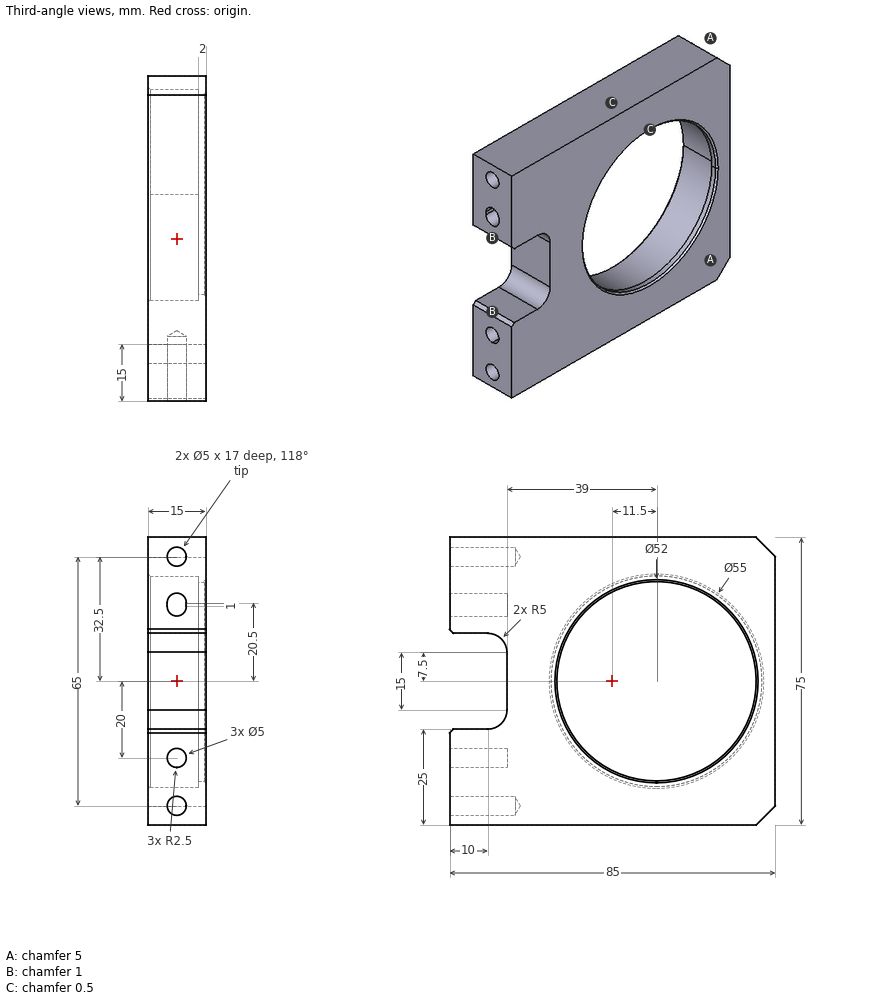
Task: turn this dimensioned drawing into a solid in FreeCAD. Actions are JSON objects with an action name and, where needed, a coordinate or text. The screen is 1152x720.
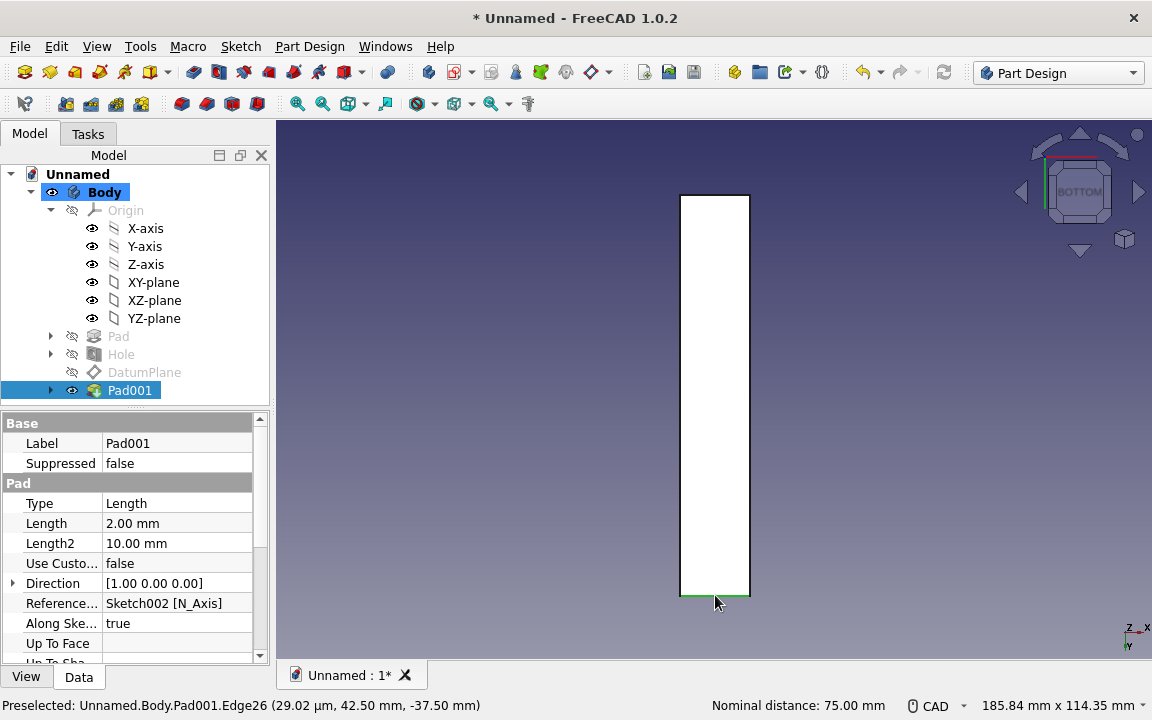
{"action": "left_click", "coordinate": [207, 104]}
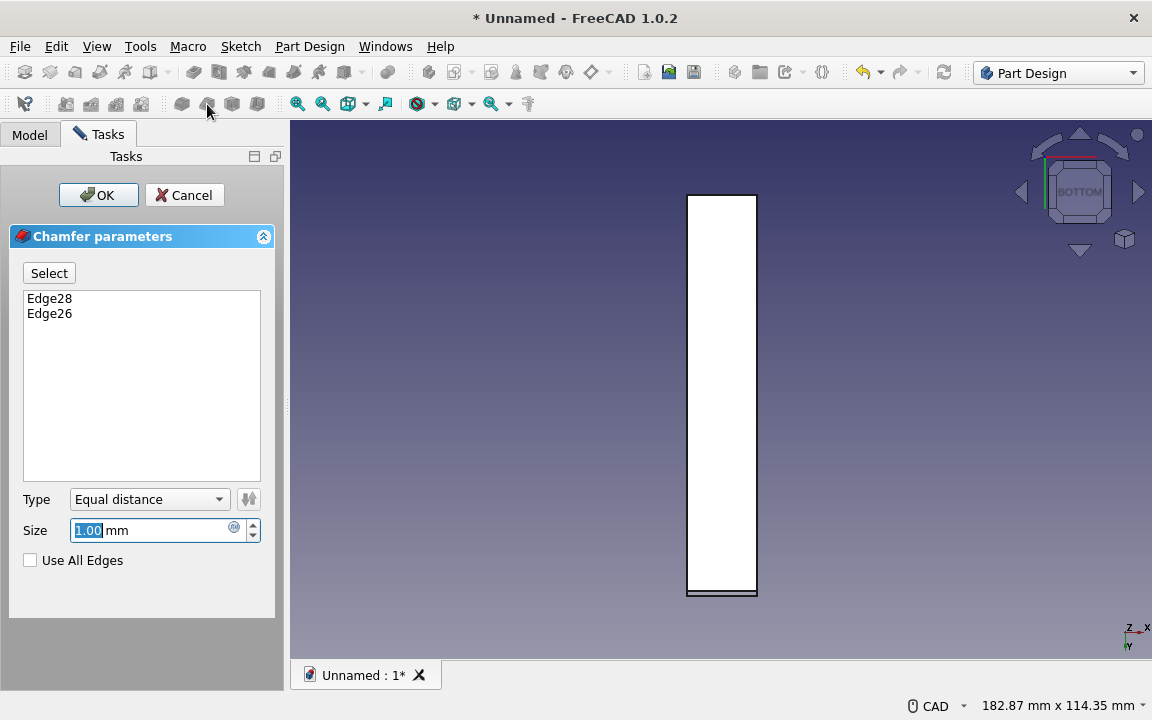
{"action": "type", "text": "5"}
{"action": "key", "text": "Tab"}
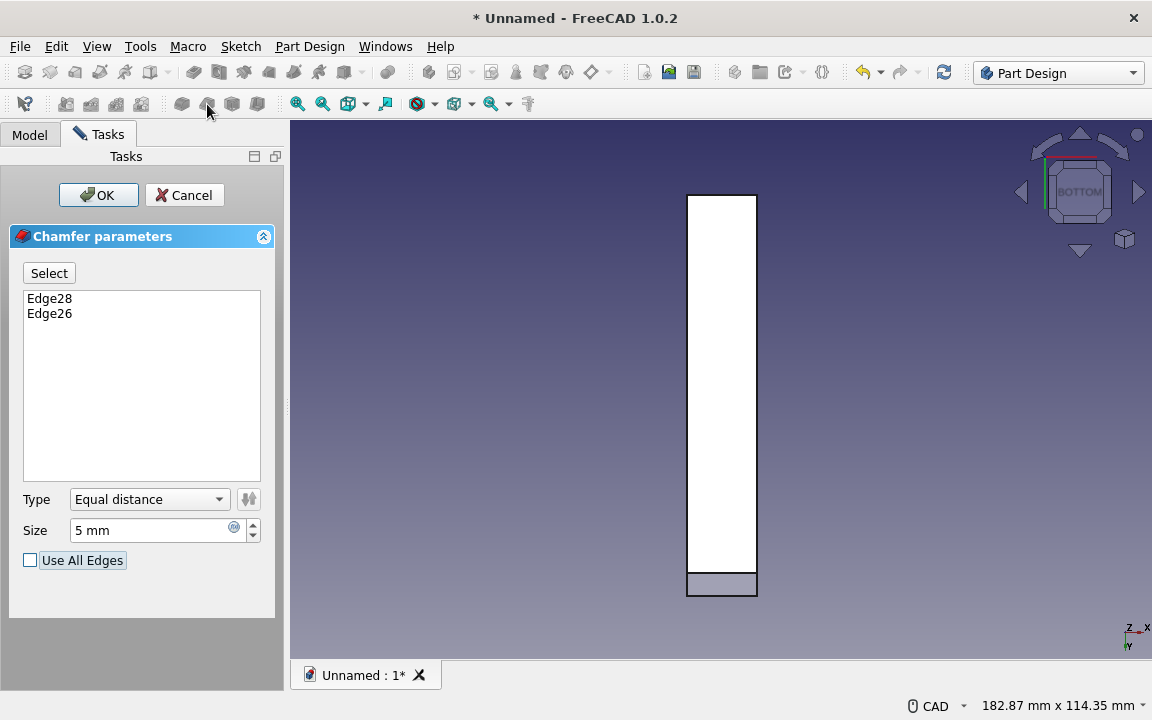
{"action": "left_click", "coordinate": [99, 195]}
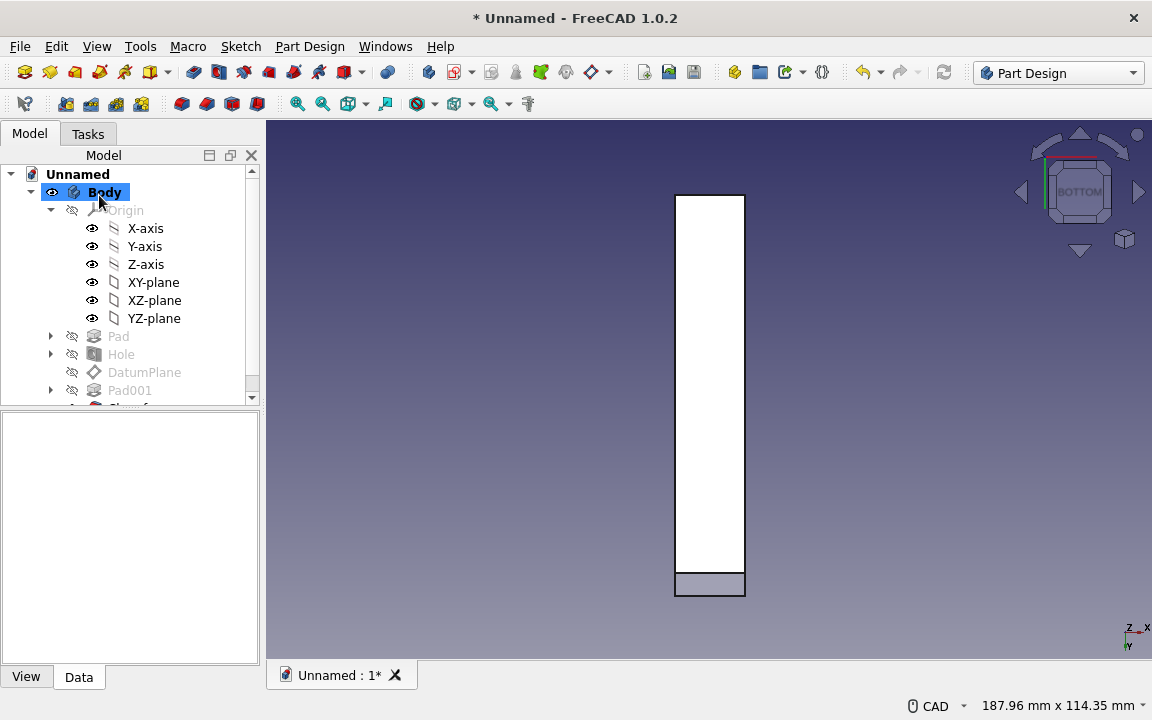
{"action": "key", "text": "0"}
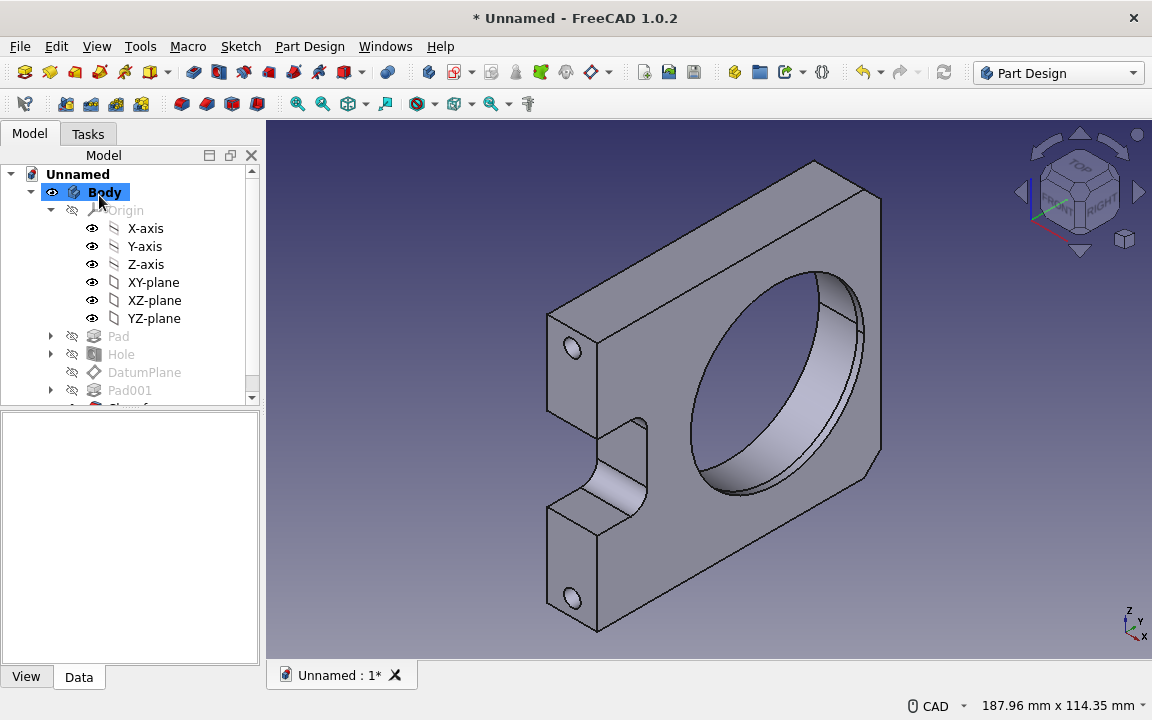
{"action": "left_click", "coordinate": [572, 555]}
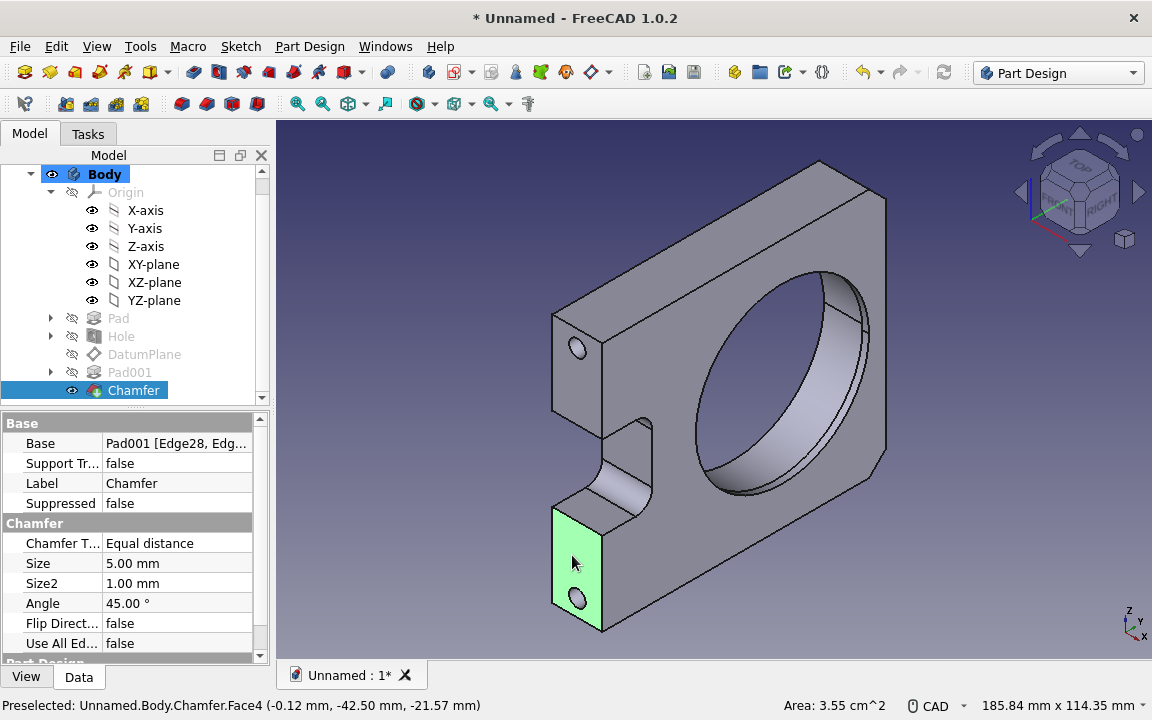
{"action": "left_click", "coordinate": [454, 72]}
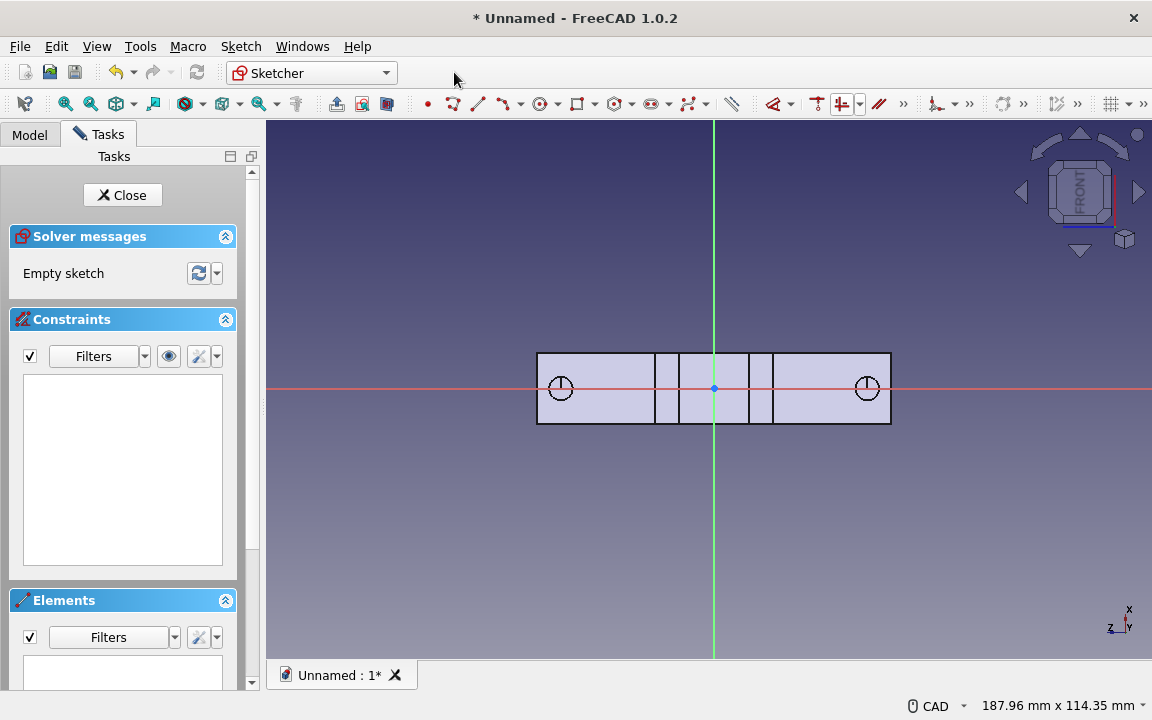
{"action": "scroll", "coordinate": [772, 388], "scroll_direction": "up", "scroll_amount": 4}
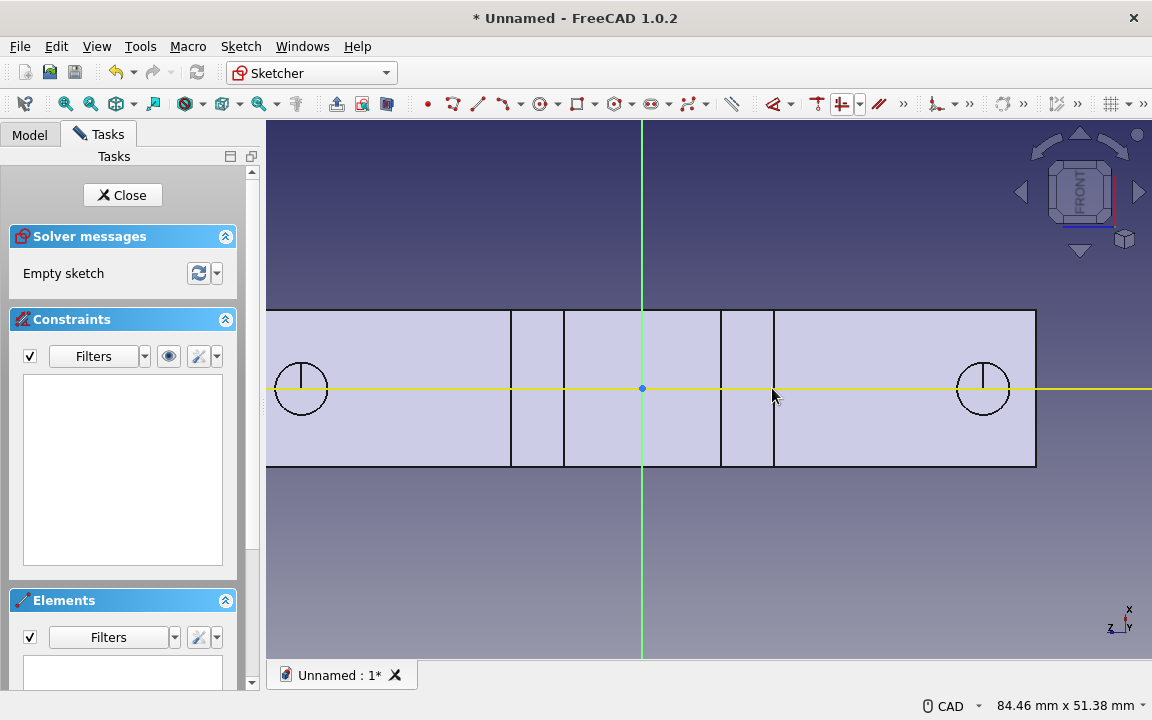
{"action": "left_click", "coordinate": [650, 104]}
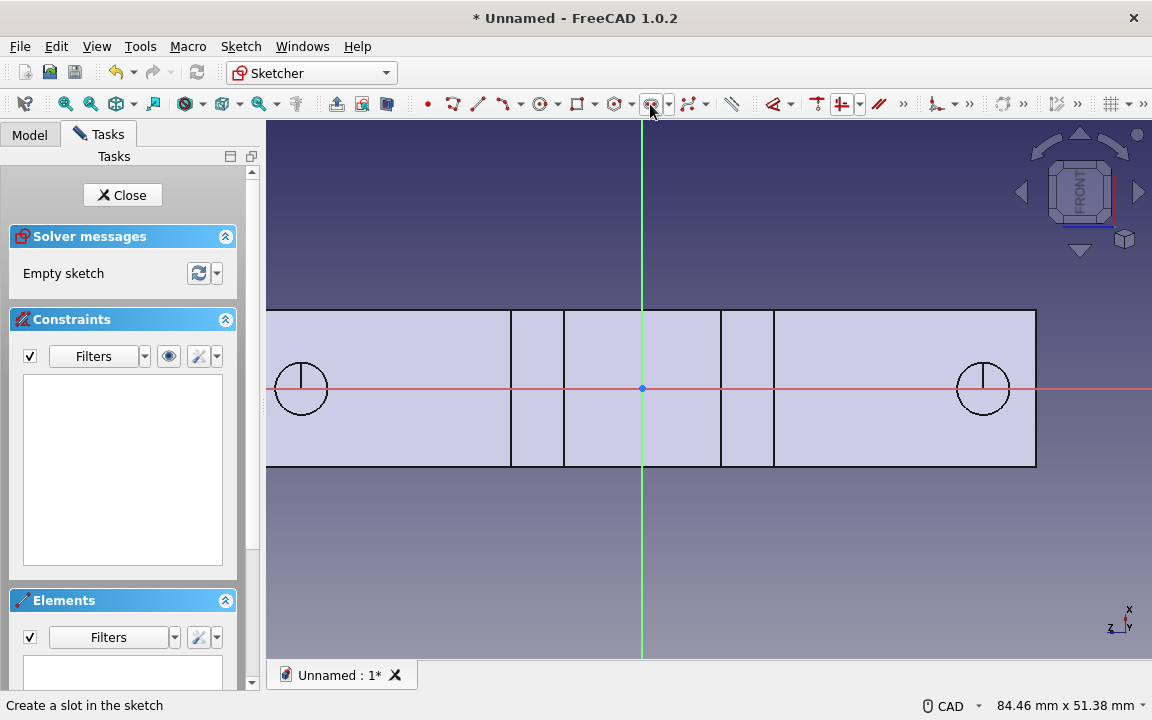
{"action": "left_click", "coordinate": [427, 389]}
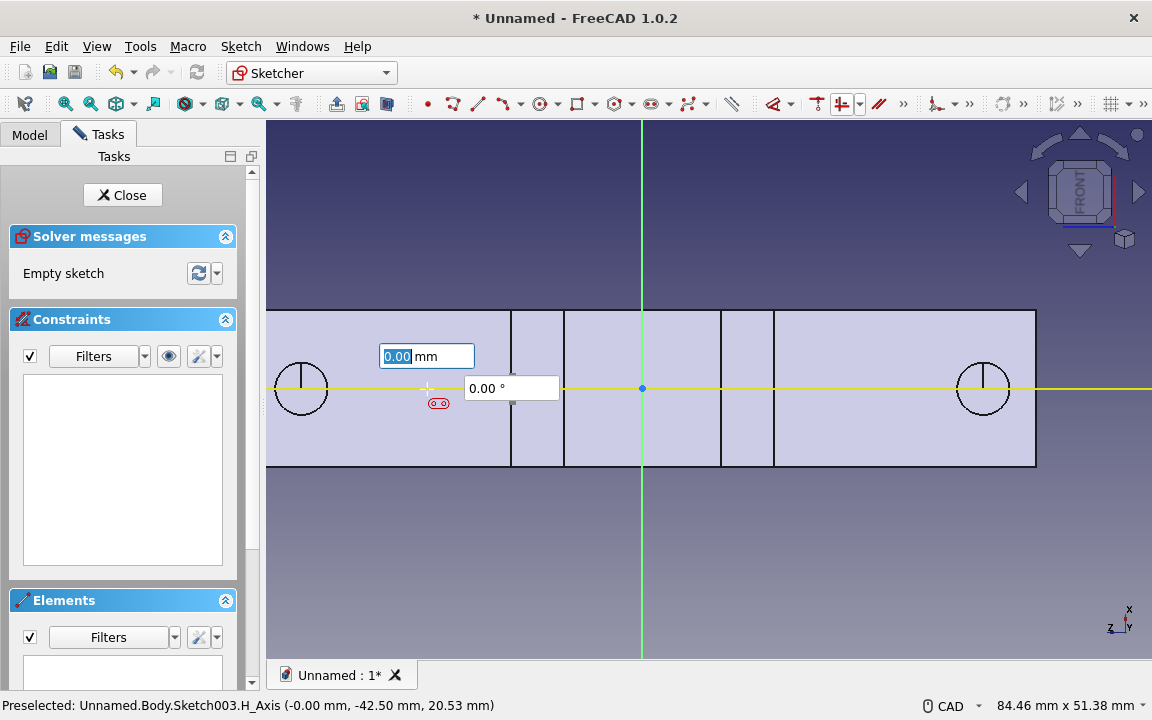
{"action": "scroll", "coordinate": [438, 389], "scroll_direction": "up", "scroll_amount": 3}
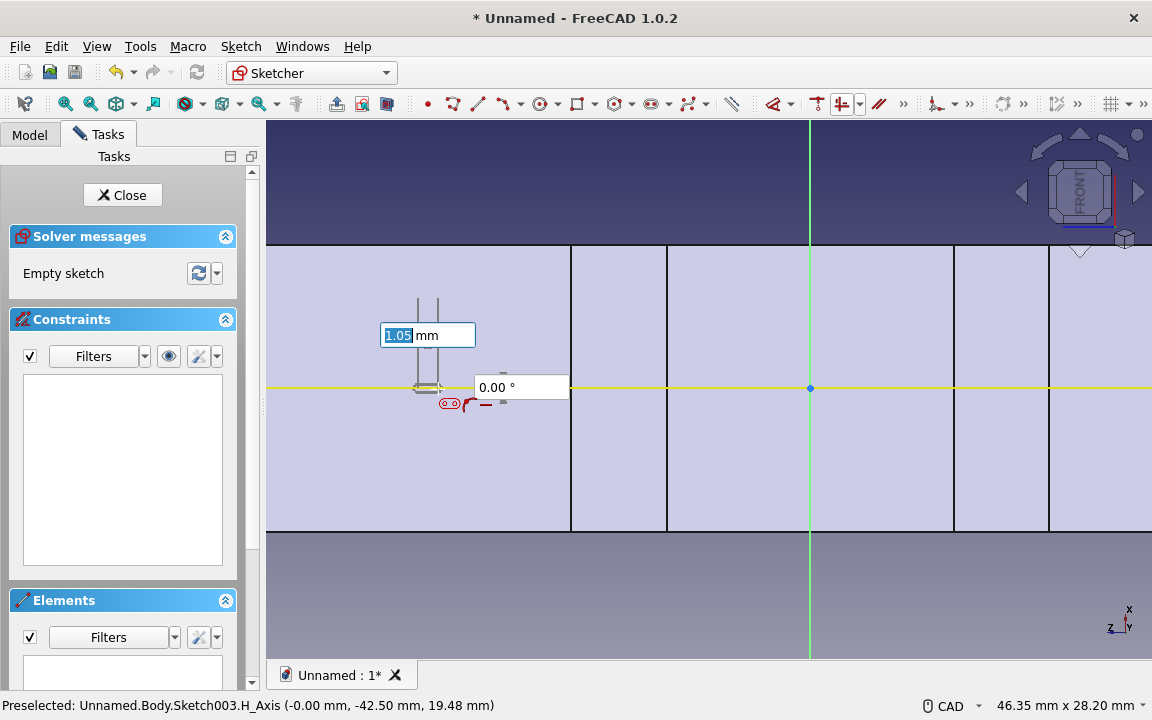
{"action": "left_click", "coordinate": [438, 379]}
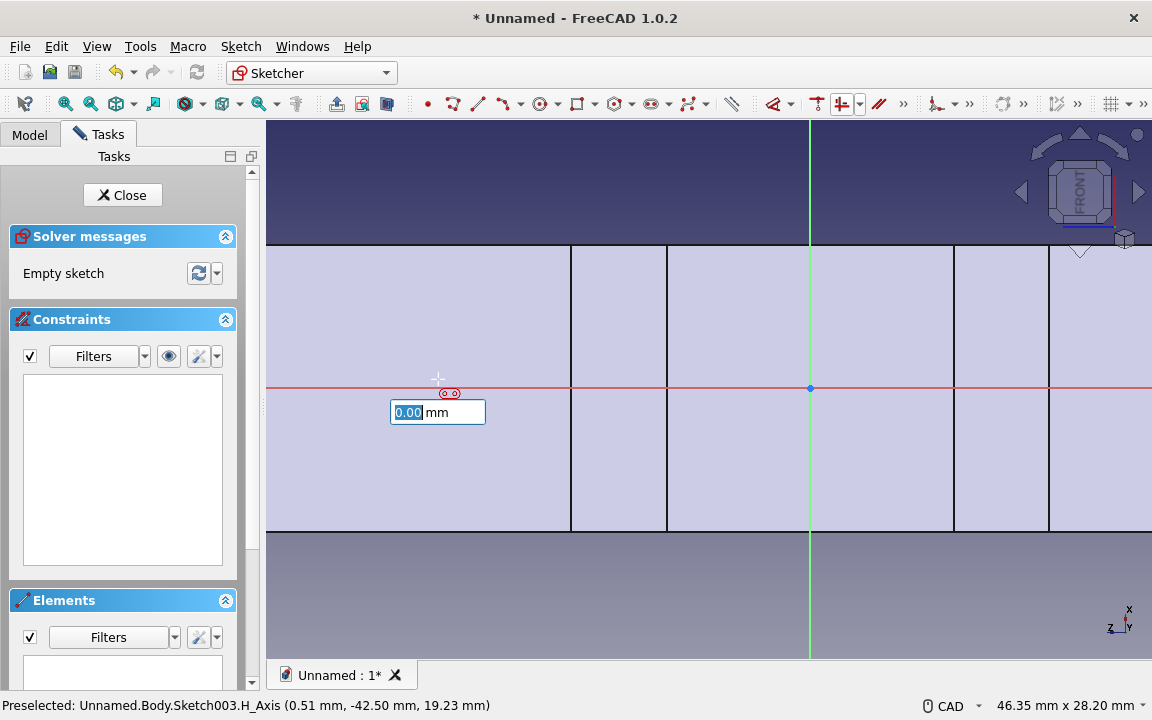
{"action": "left_click", "coordinate": [428, 340]}